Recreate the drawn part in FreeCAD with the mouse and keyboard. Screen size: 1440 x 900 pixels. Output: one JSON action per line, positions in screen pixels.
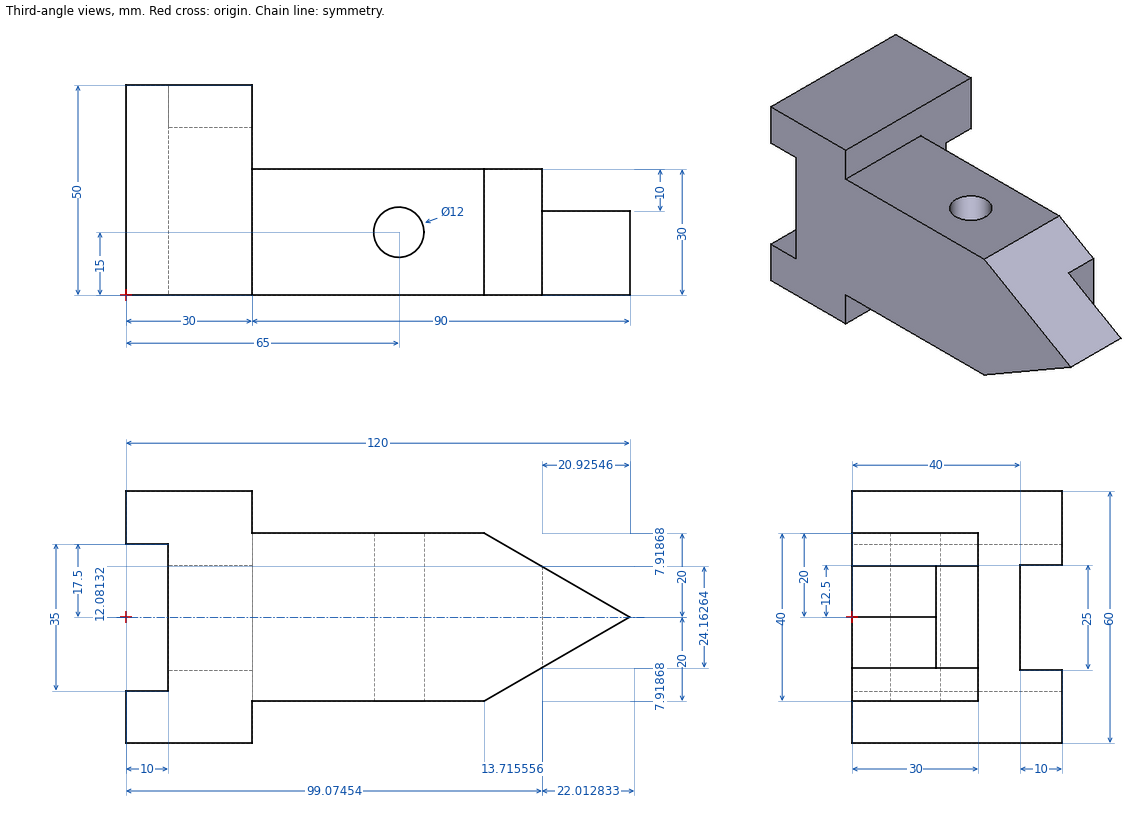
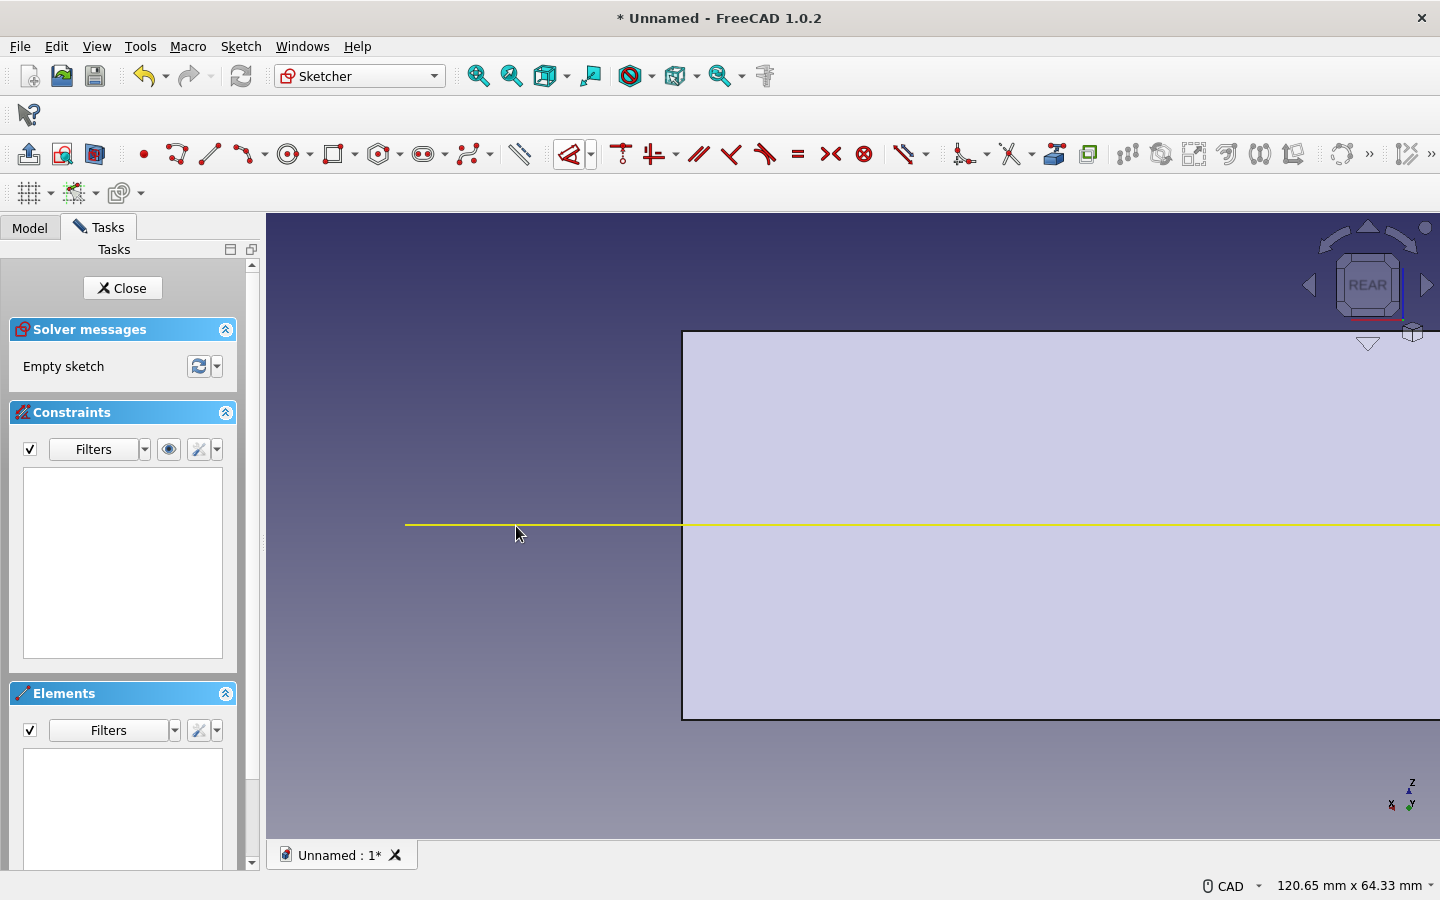
{"action": "left_click", "coordinate": [177, 154]}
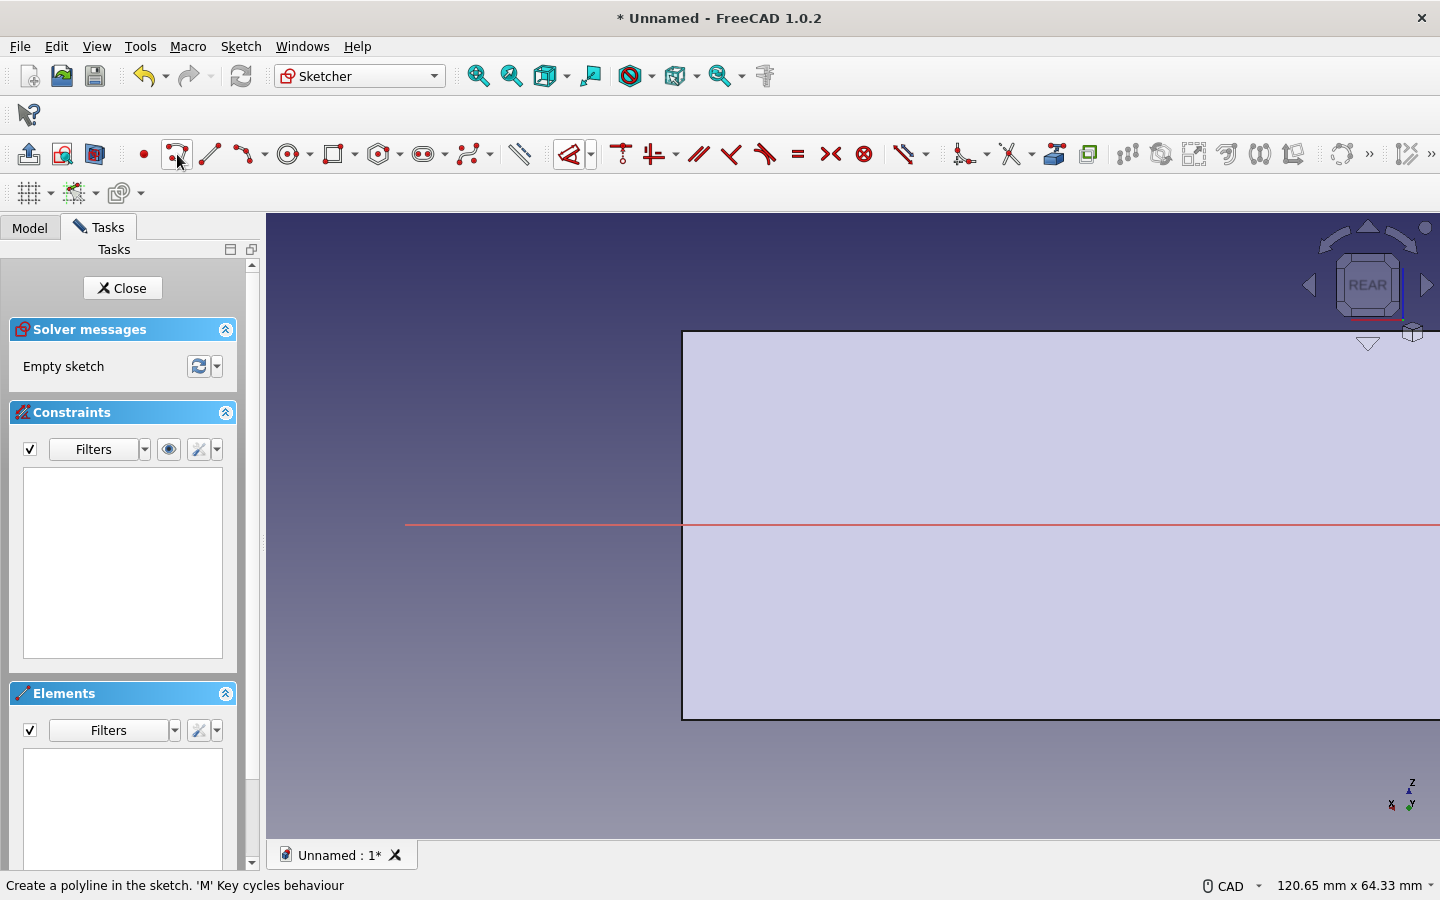
{"action": "left_click", "coordinate": [886, 408]}
{"action": "left_click", "coordinate": [886, 331]}
{"action": "left_click", "coordinate": [682, 331]}
{"action": "left_click", "coordinate": [682, 525]}
{"action": "left_click", "coordinate": [886, 409]}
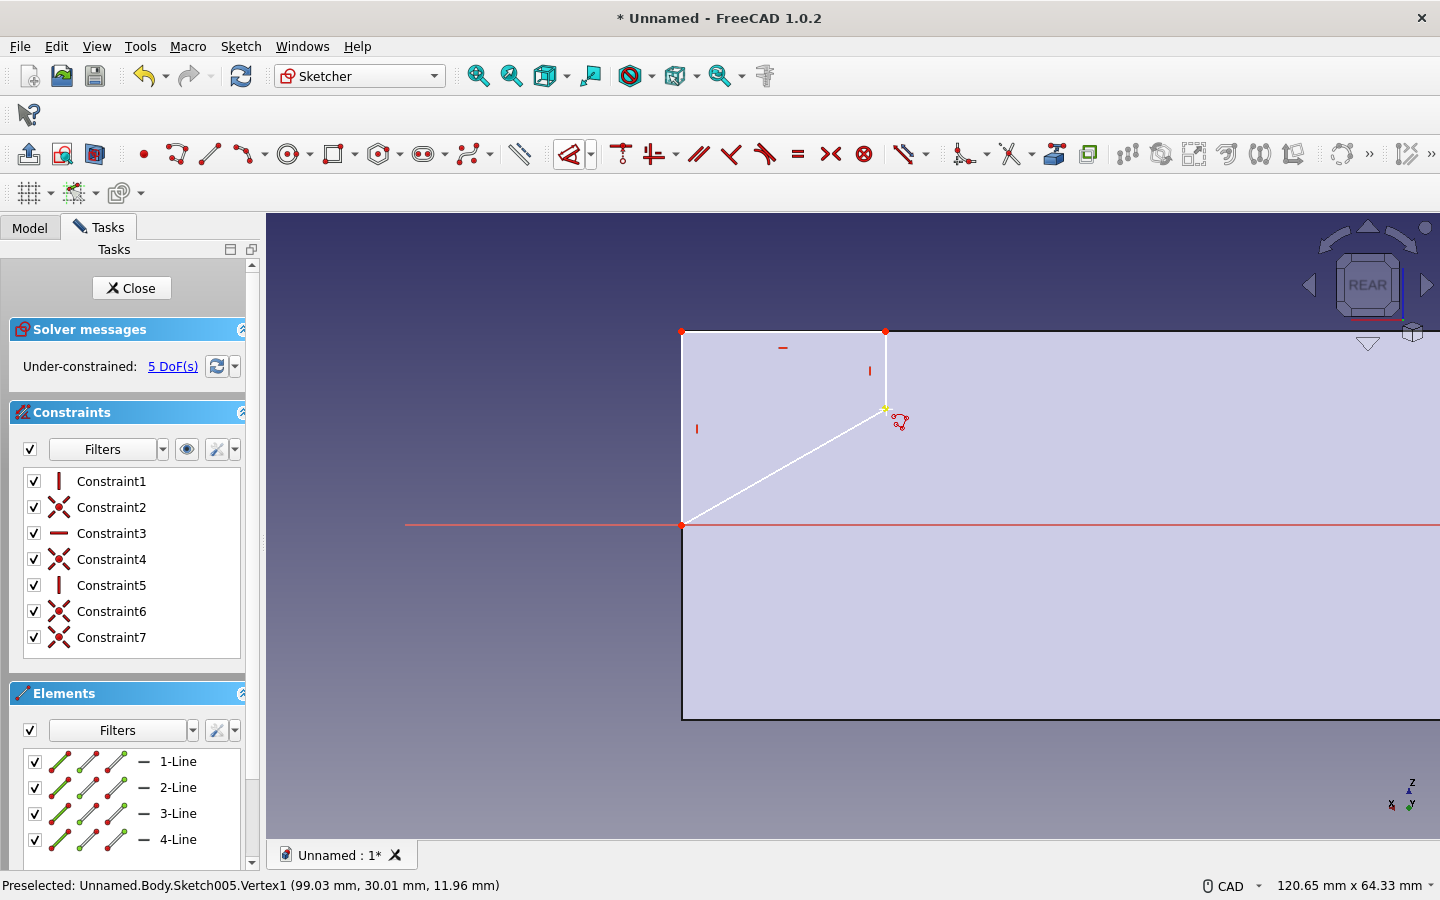
{"action": "left_click", "coordinate": [886, 643]}
{"action": "left_click", "coordinate": [682, 525]}
{"action": "left_click", "coordinate": [682, 720]}
{"action": "left_click", "coordinate": [886, 720]}
{"action": "left_click", "coordinate": [886, 644]}
{"action": "key", "text": "Escape"}
{"action": "key", "text": "Escape"}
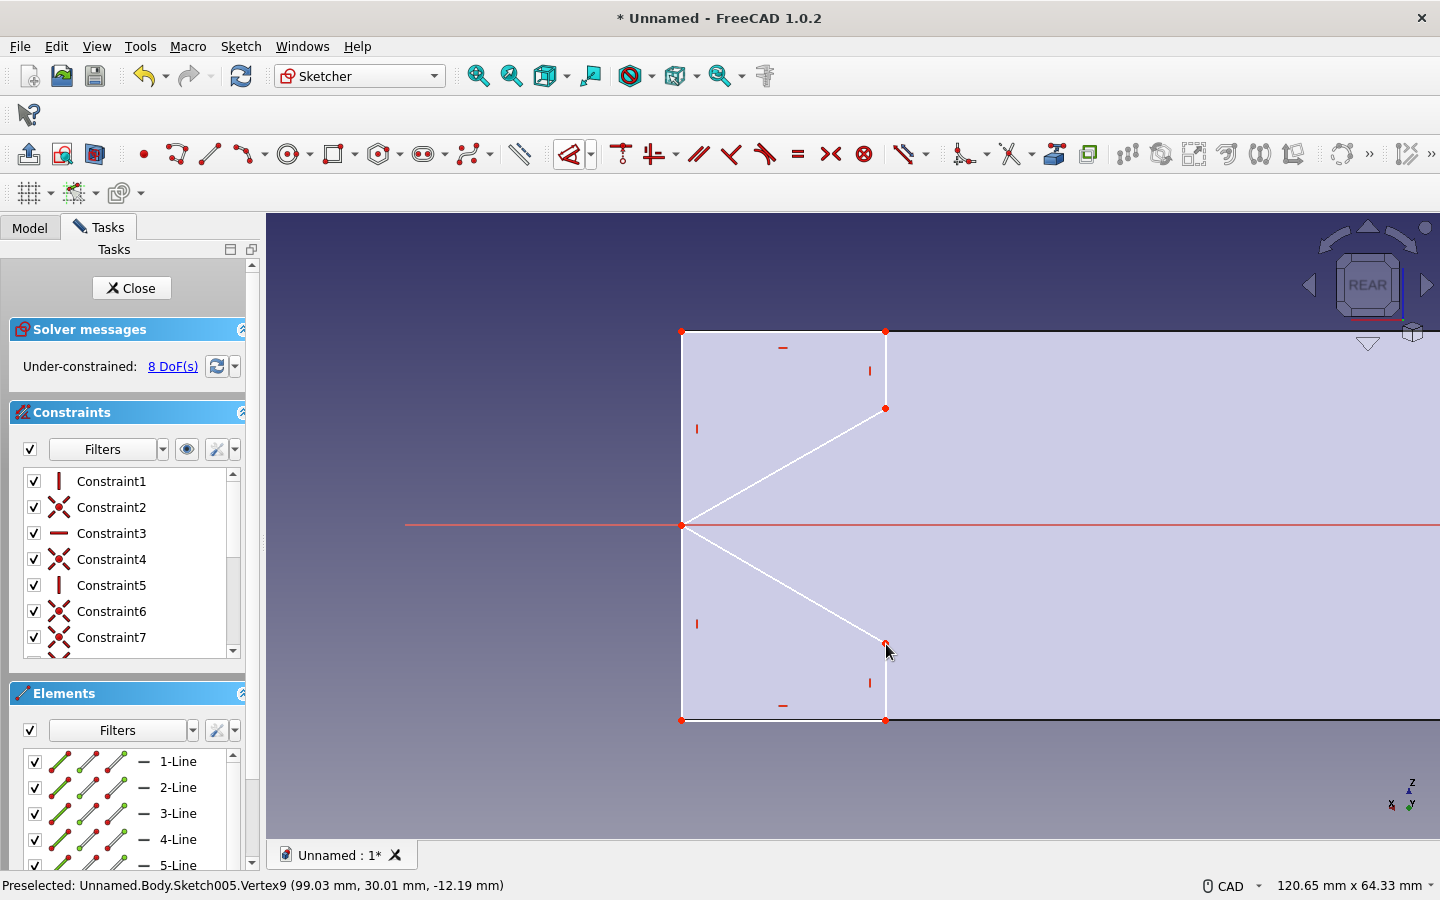
{"action": "left_click", "coordinate": [886, 409]}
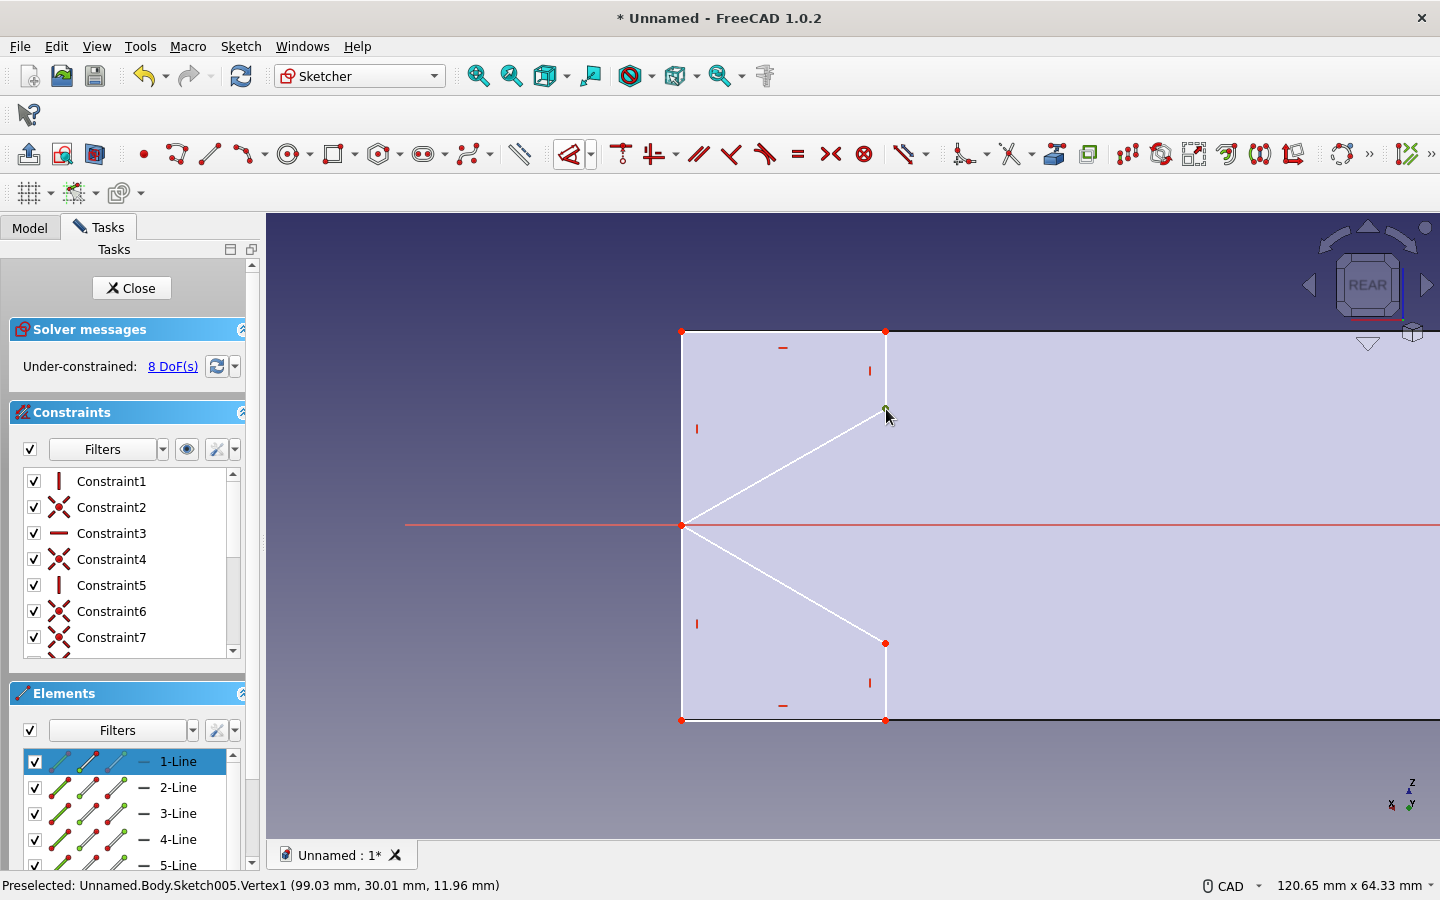
{"action": "left_click", "coordinate": [886, 644]}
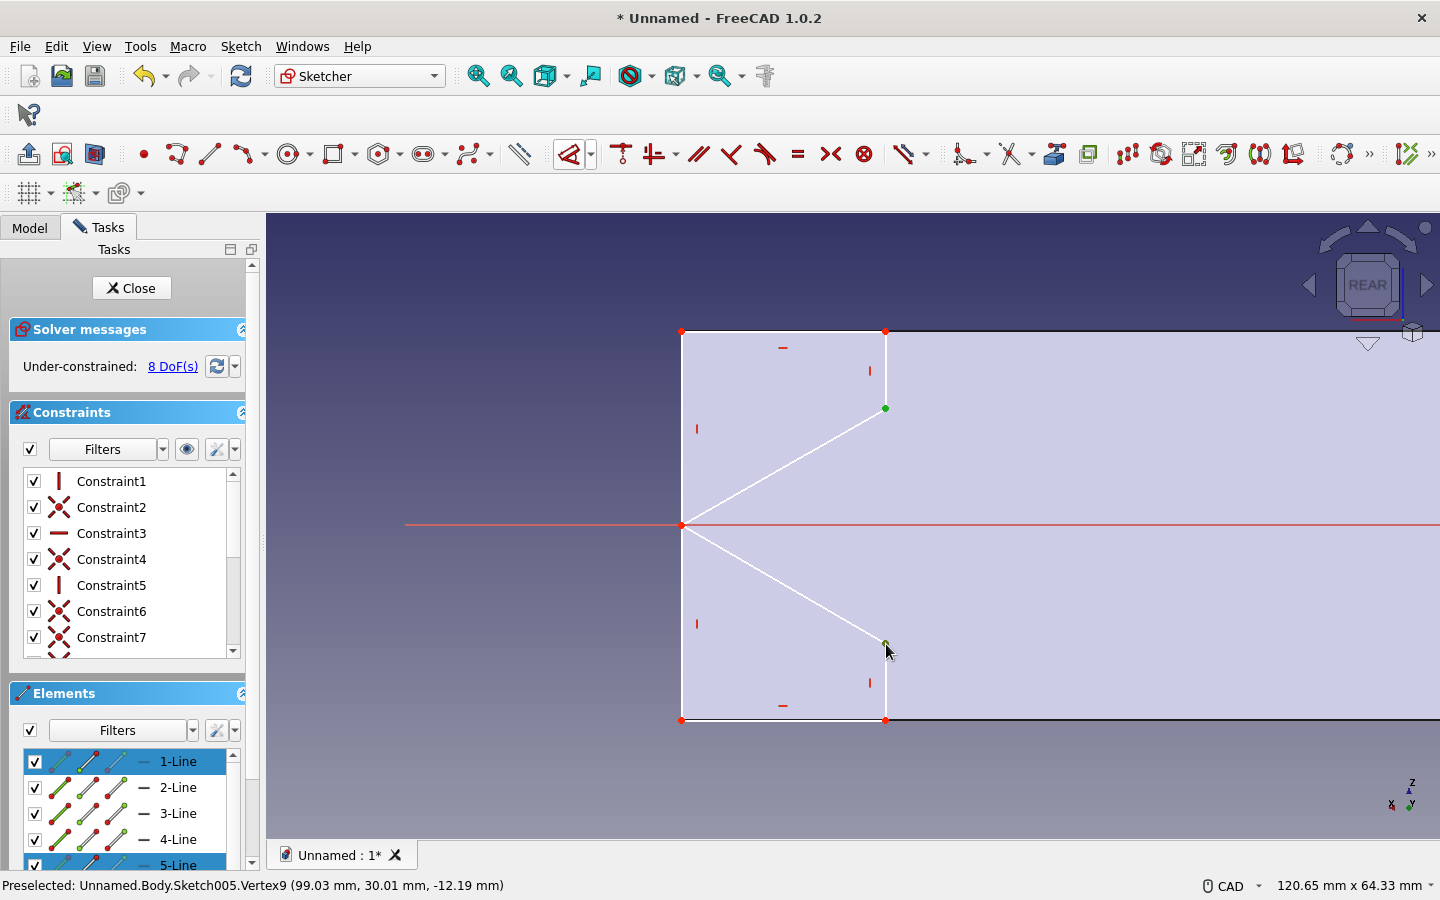
{"action": "left_click", "coordinate": [434, 525]}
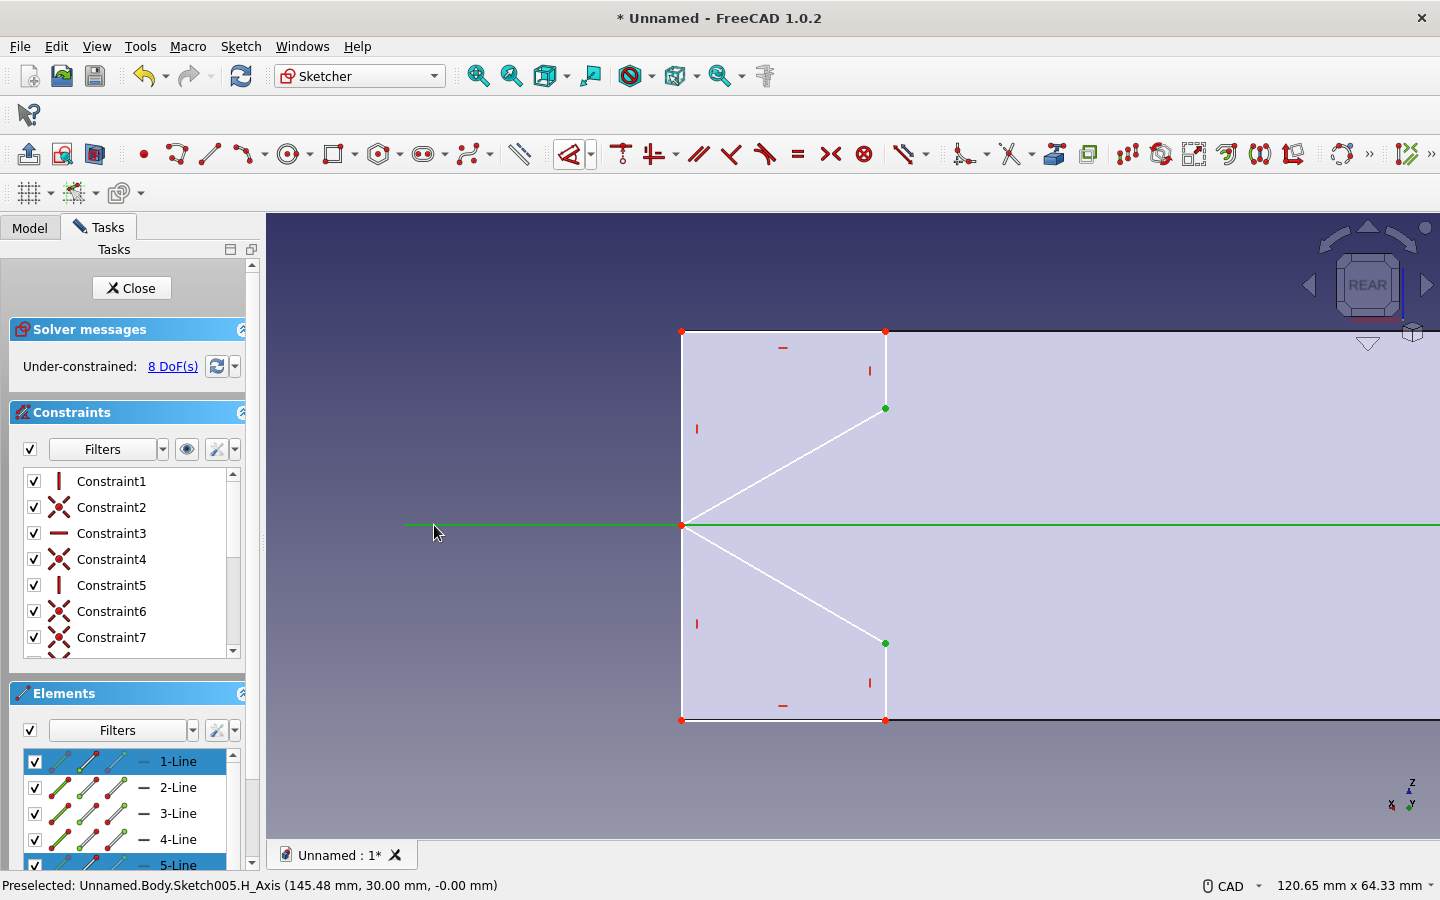
{"action": "left_click", "coordinate": [831, 154]}